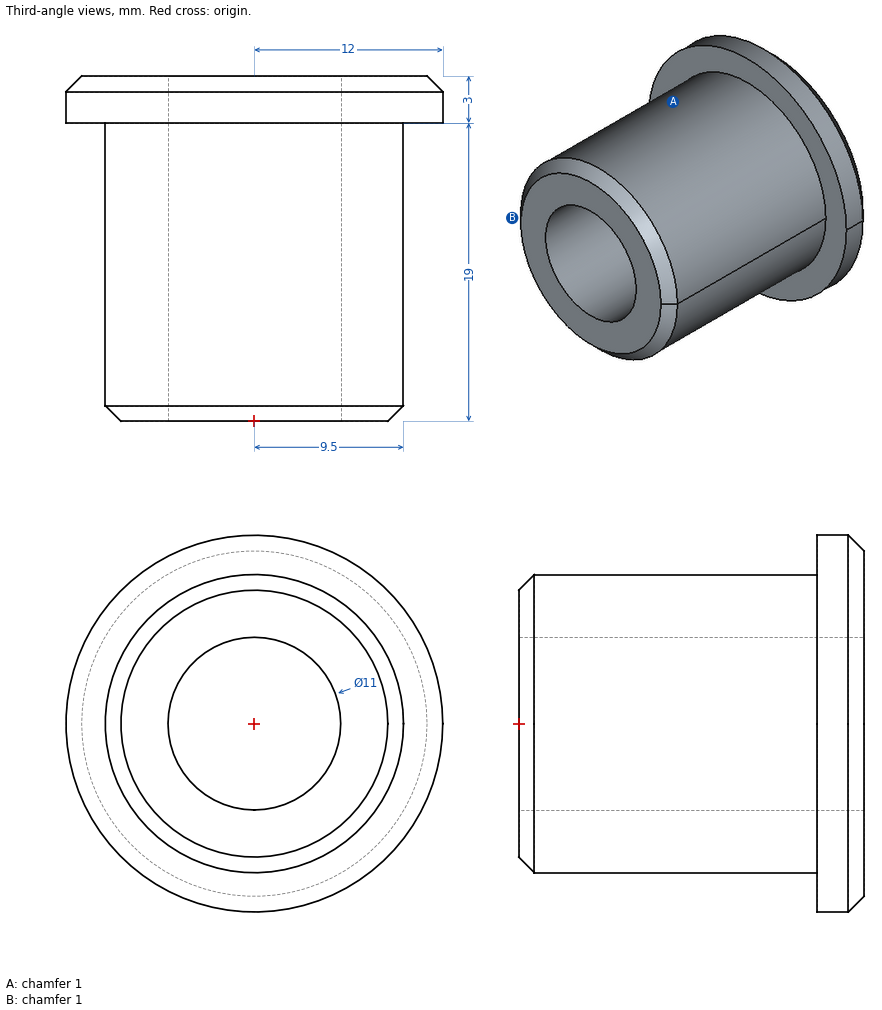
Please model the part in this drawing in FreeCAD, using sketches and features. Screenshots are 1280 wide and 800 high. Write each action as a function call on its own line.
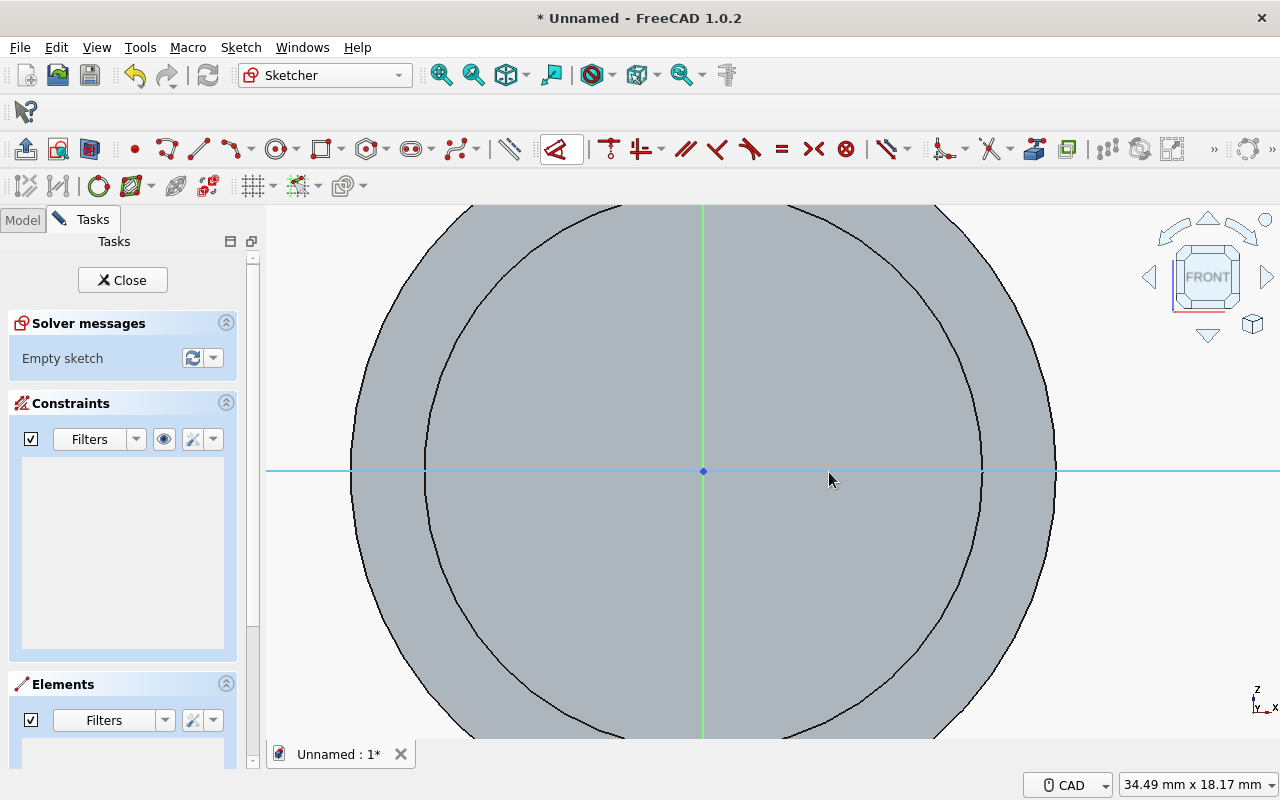
click(276, 150)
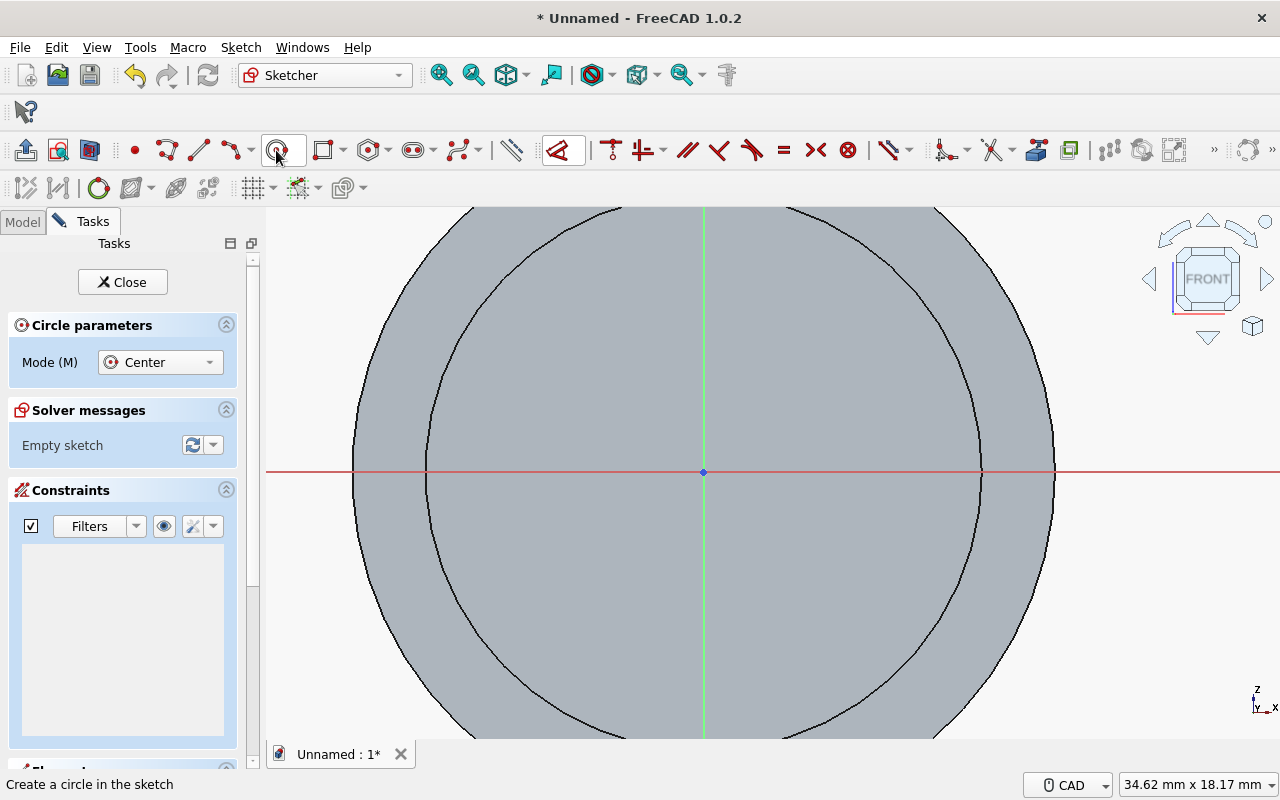
click(704, 472)
click(818, 358)
key(Escape)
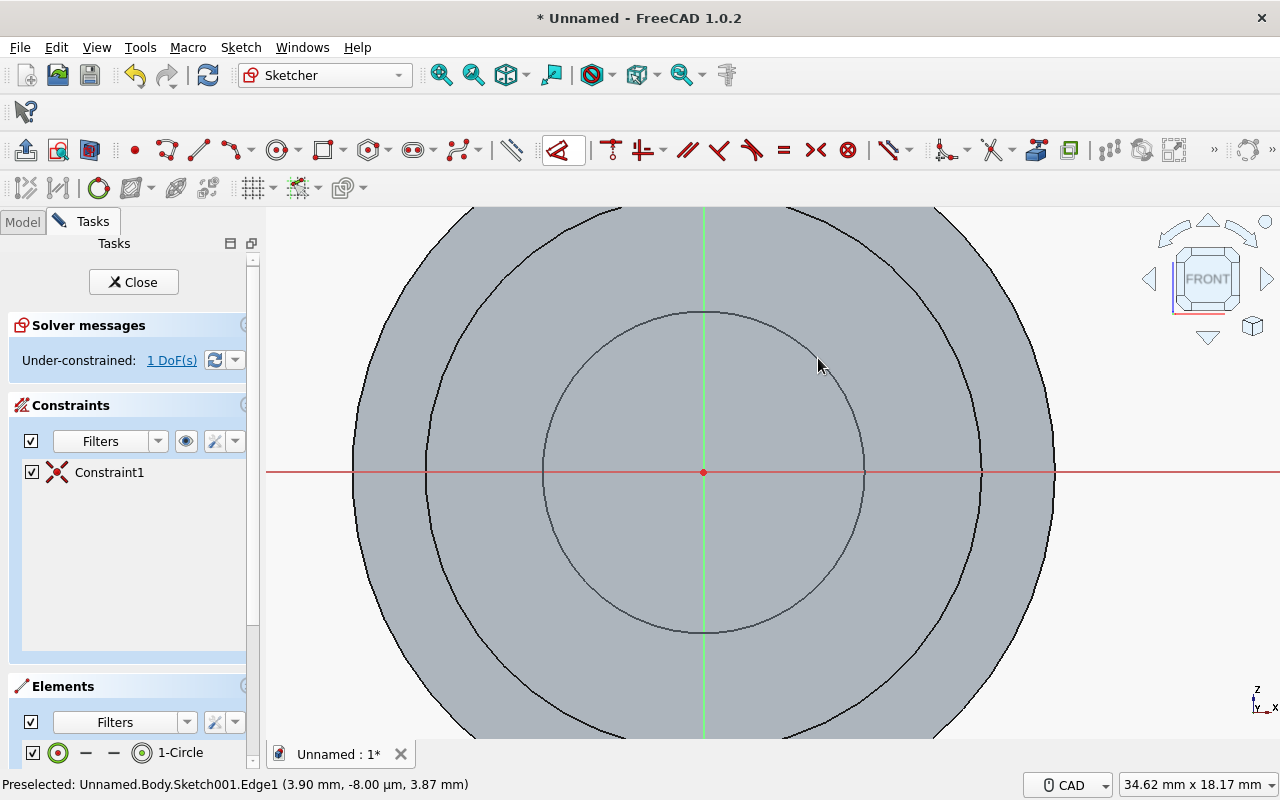
click(817, 358)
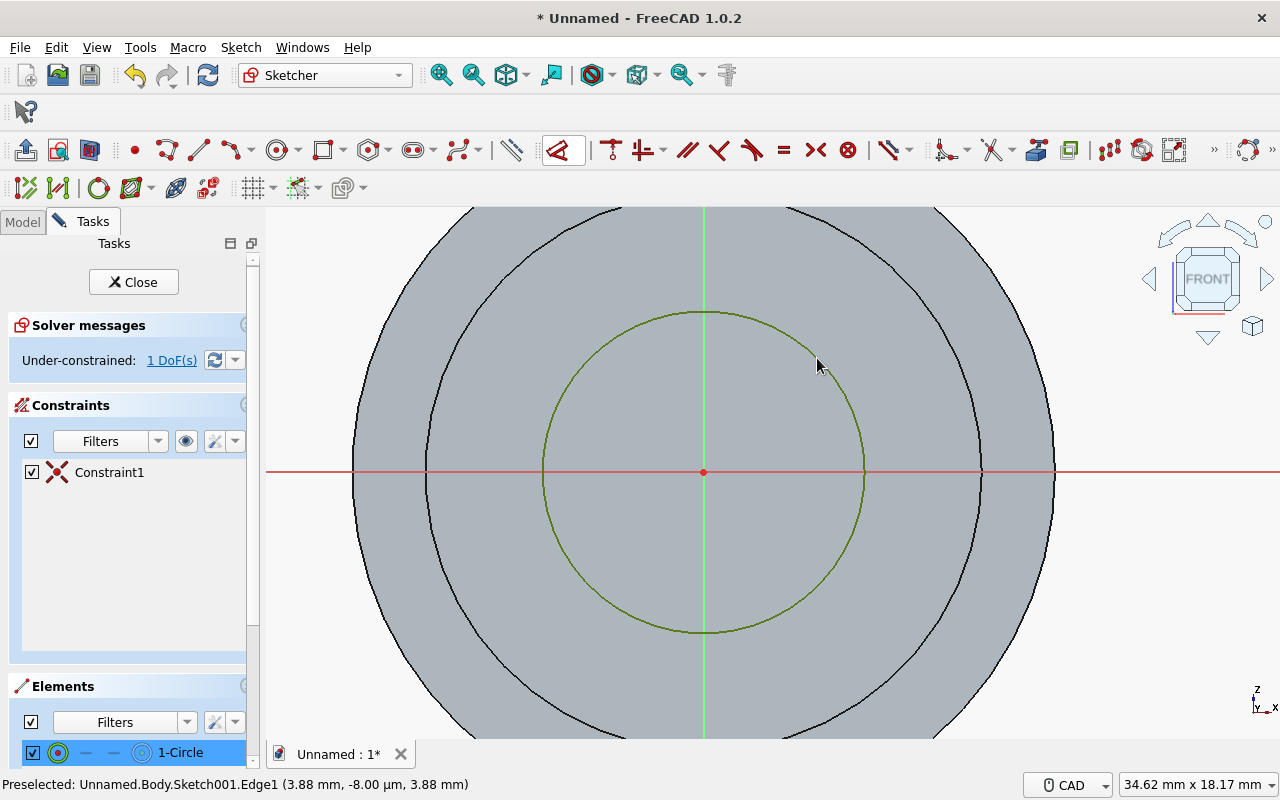
key(k)
key(o)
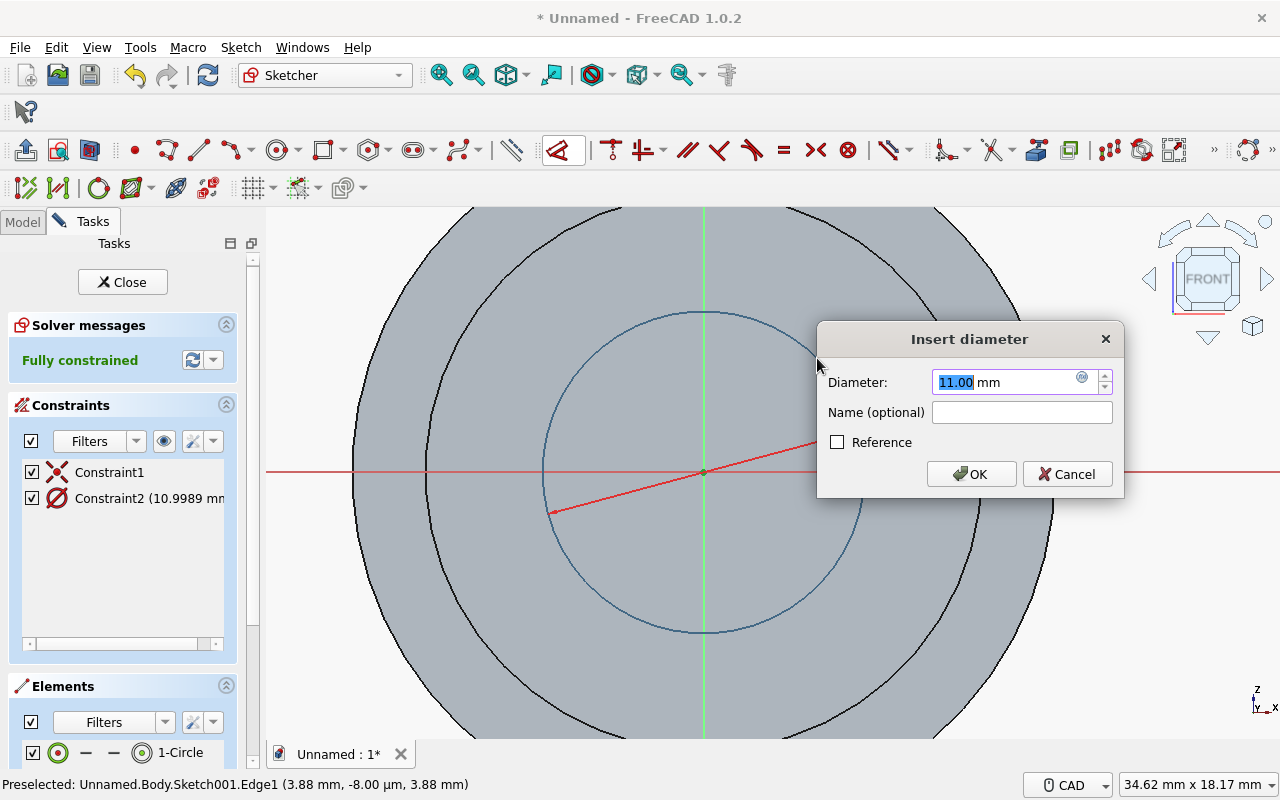
text(11)
key(Return)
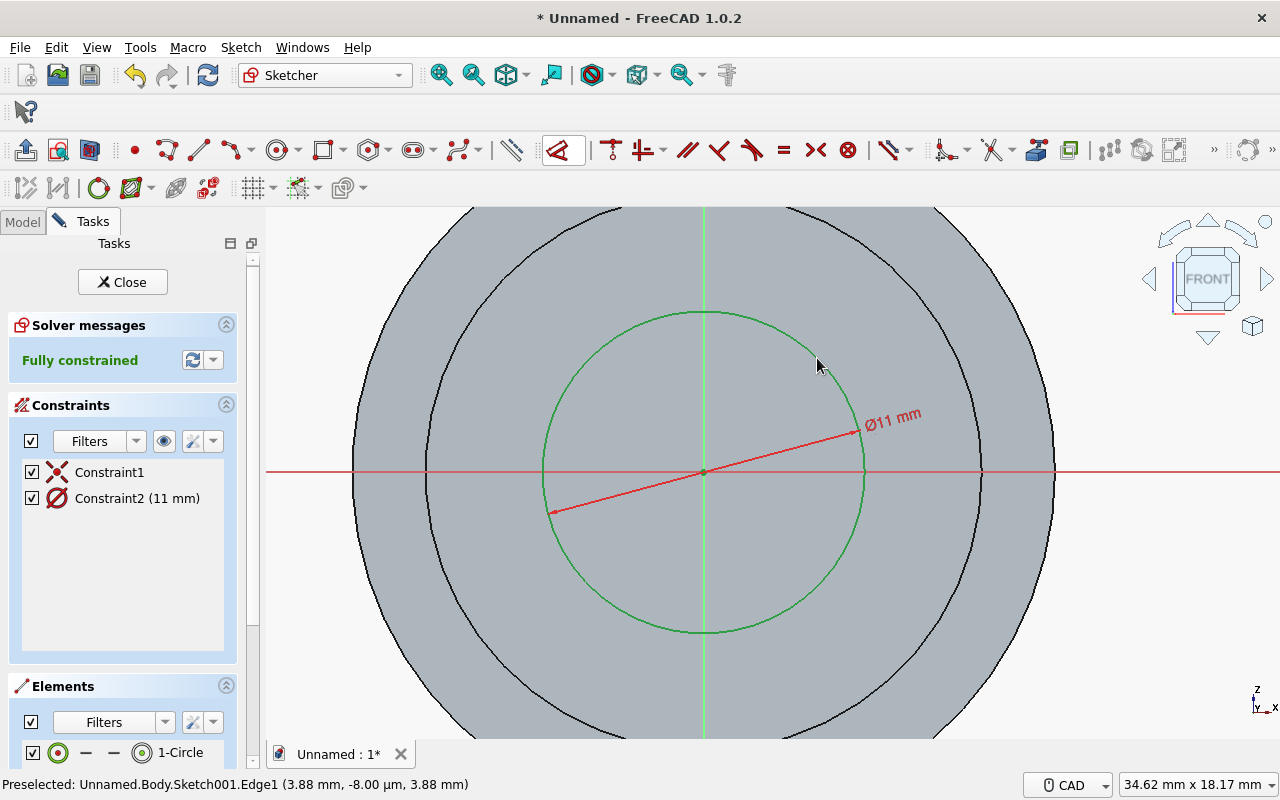
click(123, 282)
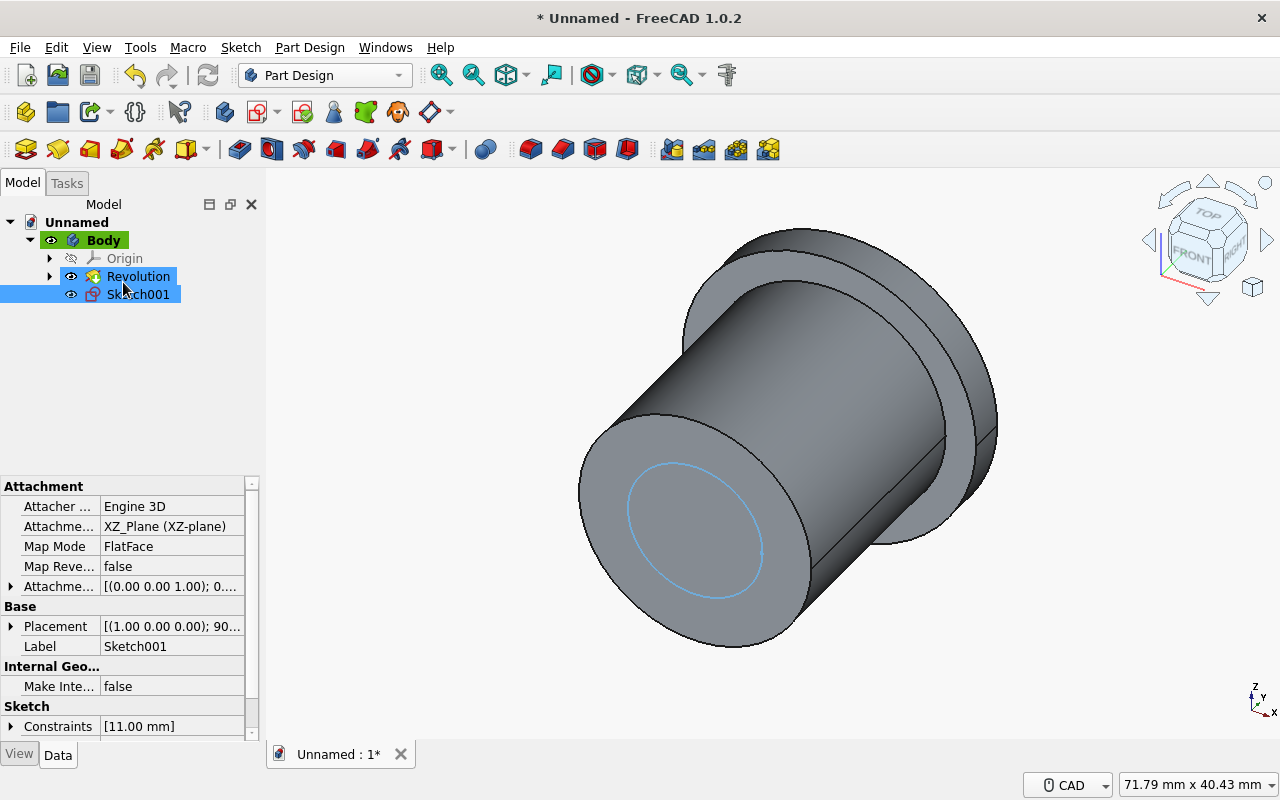
click(240, 150)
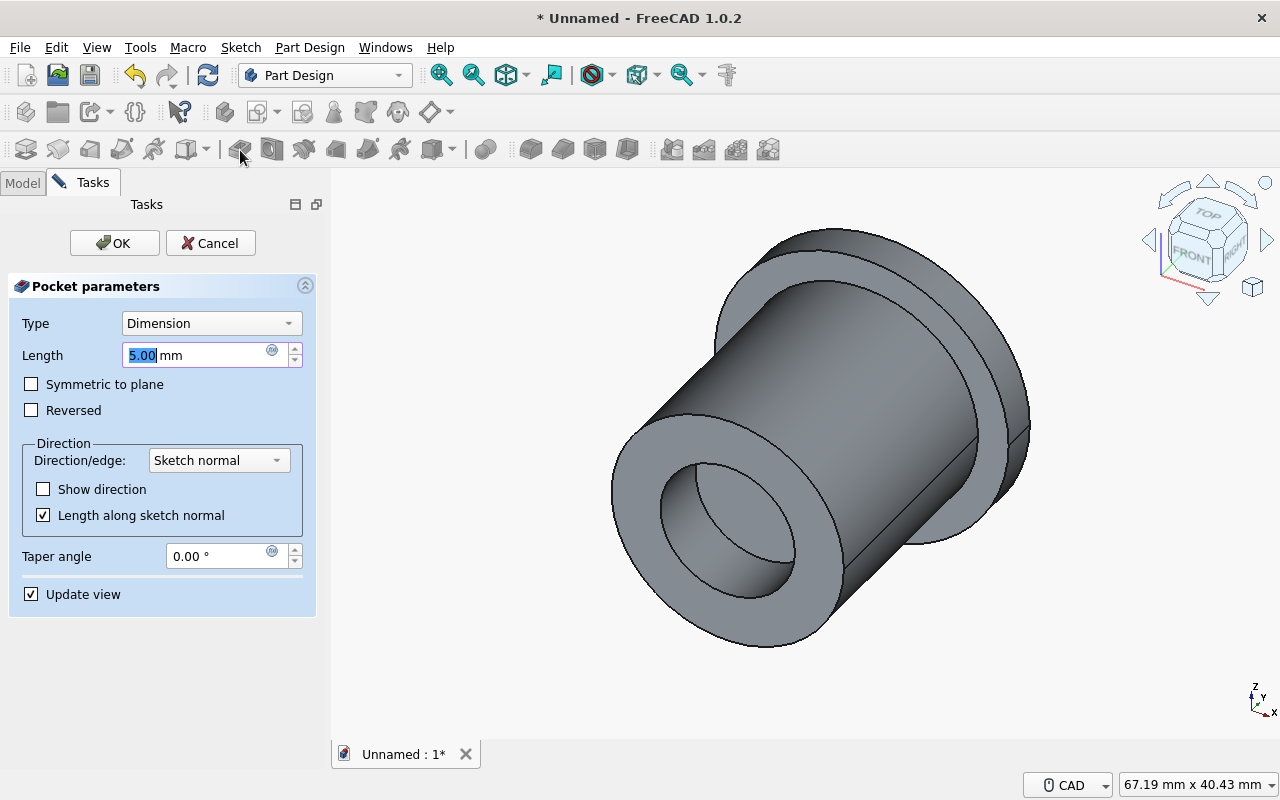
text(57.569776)
key(Tab)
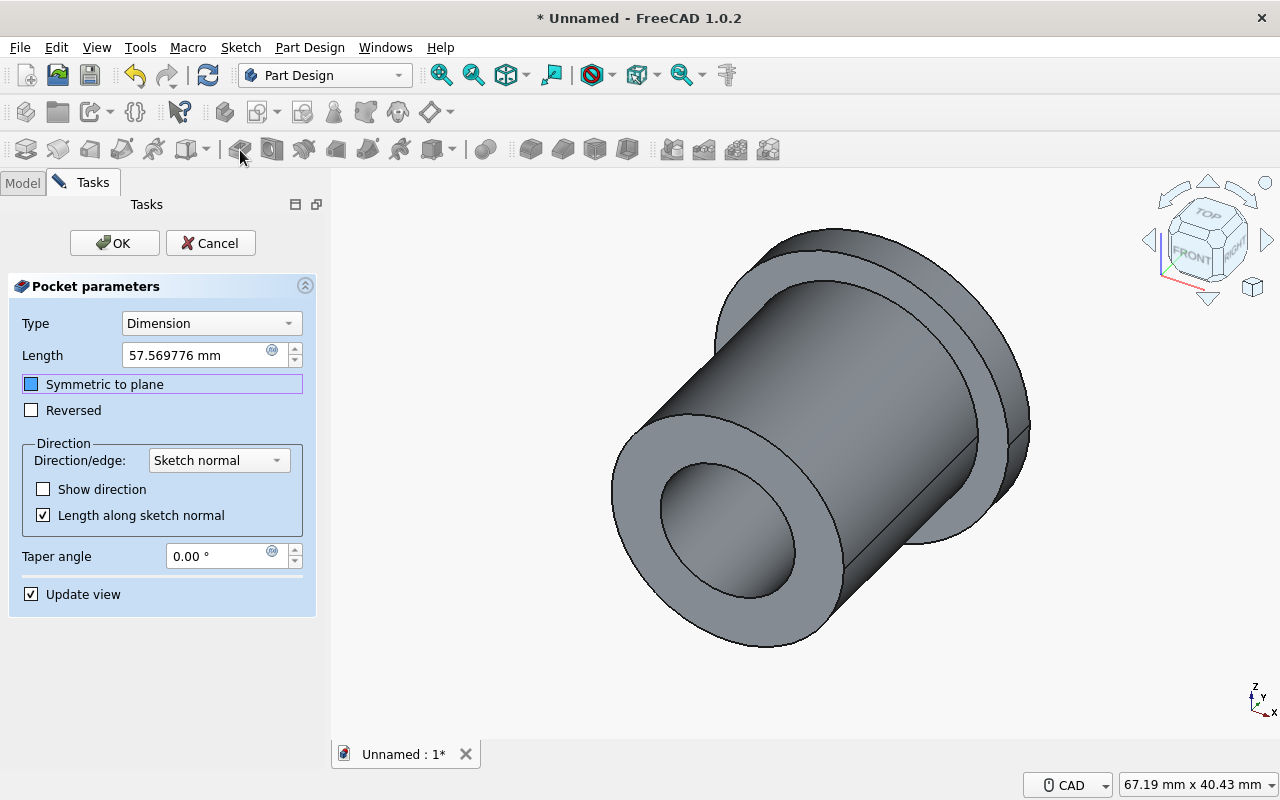
click(30, 384)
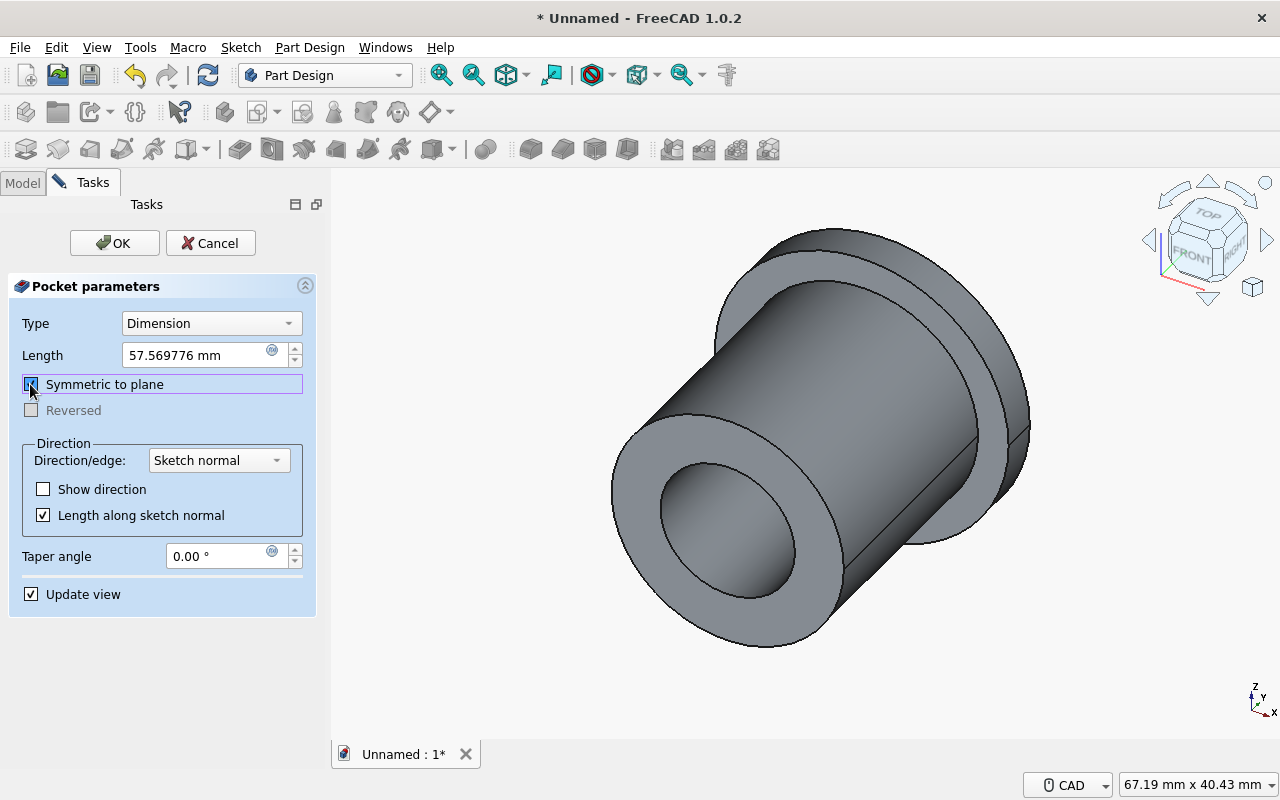
click(115, 243)